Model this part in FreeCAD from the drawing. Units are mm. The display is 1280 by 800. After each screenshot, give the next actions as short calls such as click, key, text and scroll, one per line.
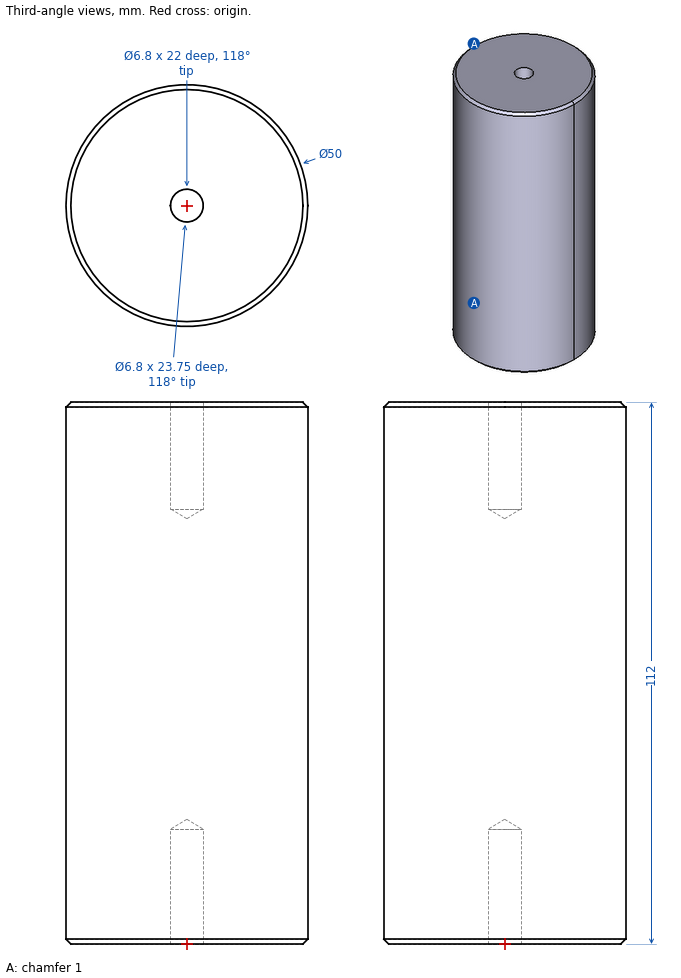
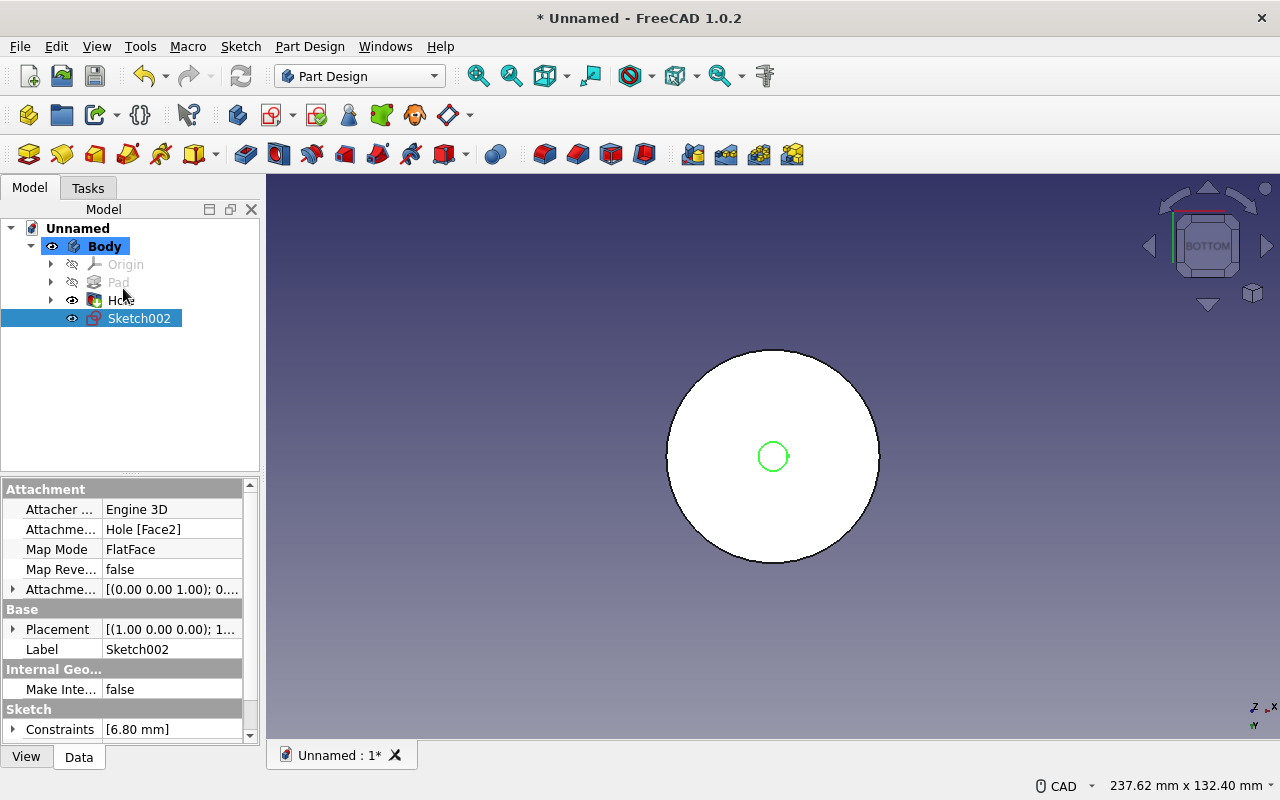
click(279, 154)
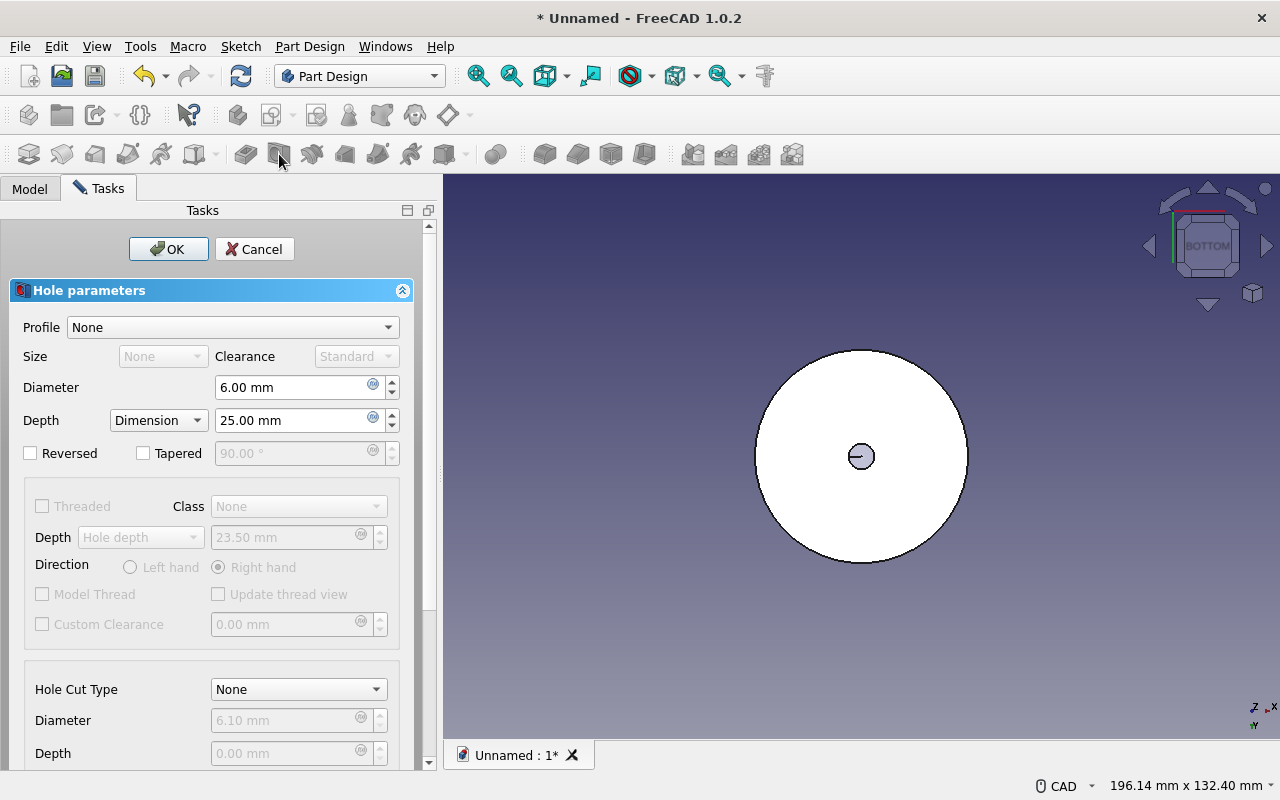
triple_click(300, 388)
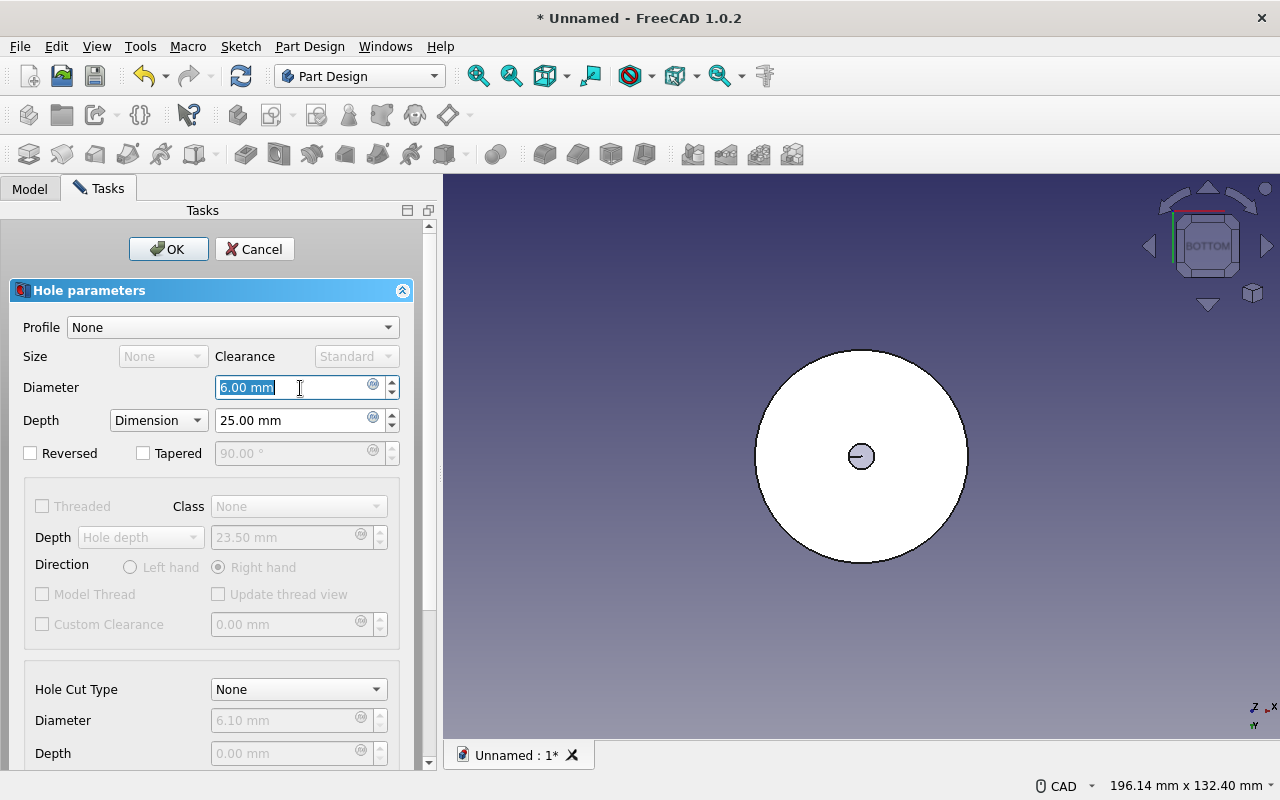
text(6.8)
key(Tab)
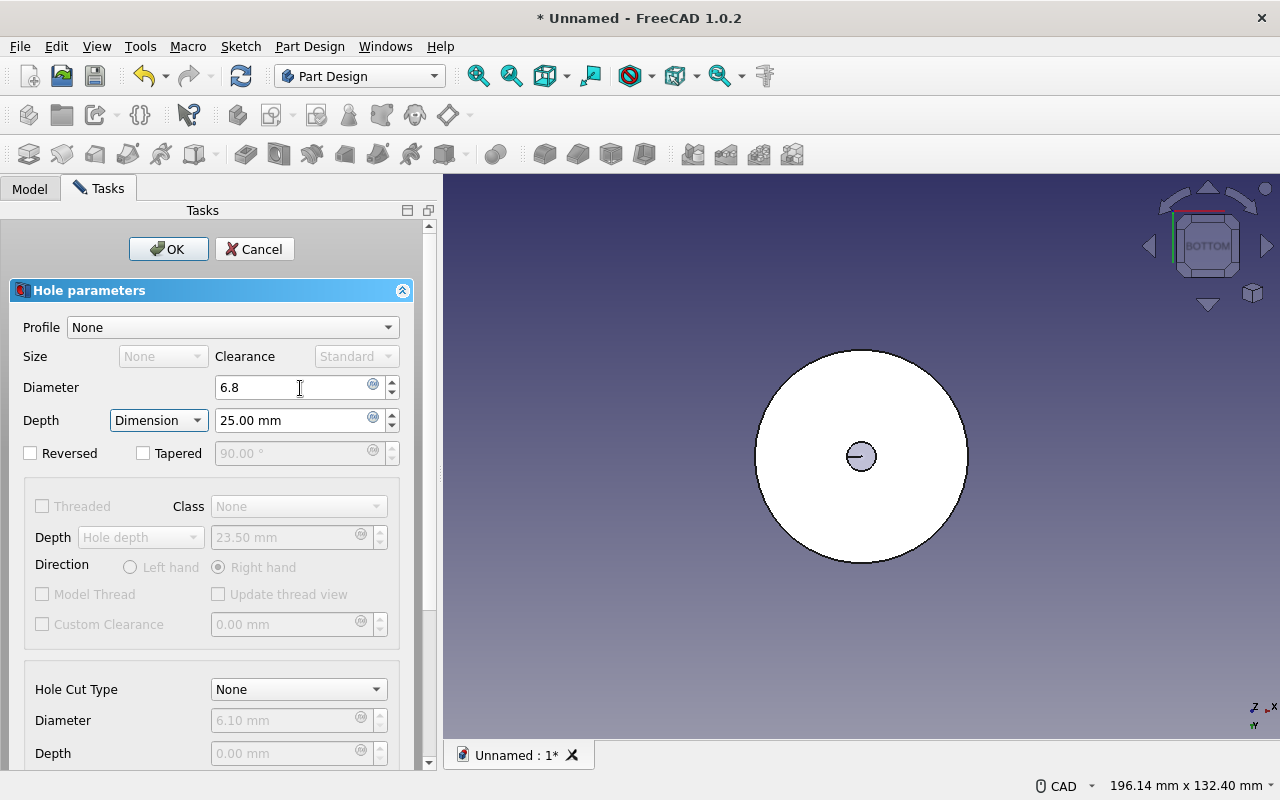
triple_click(300, 420)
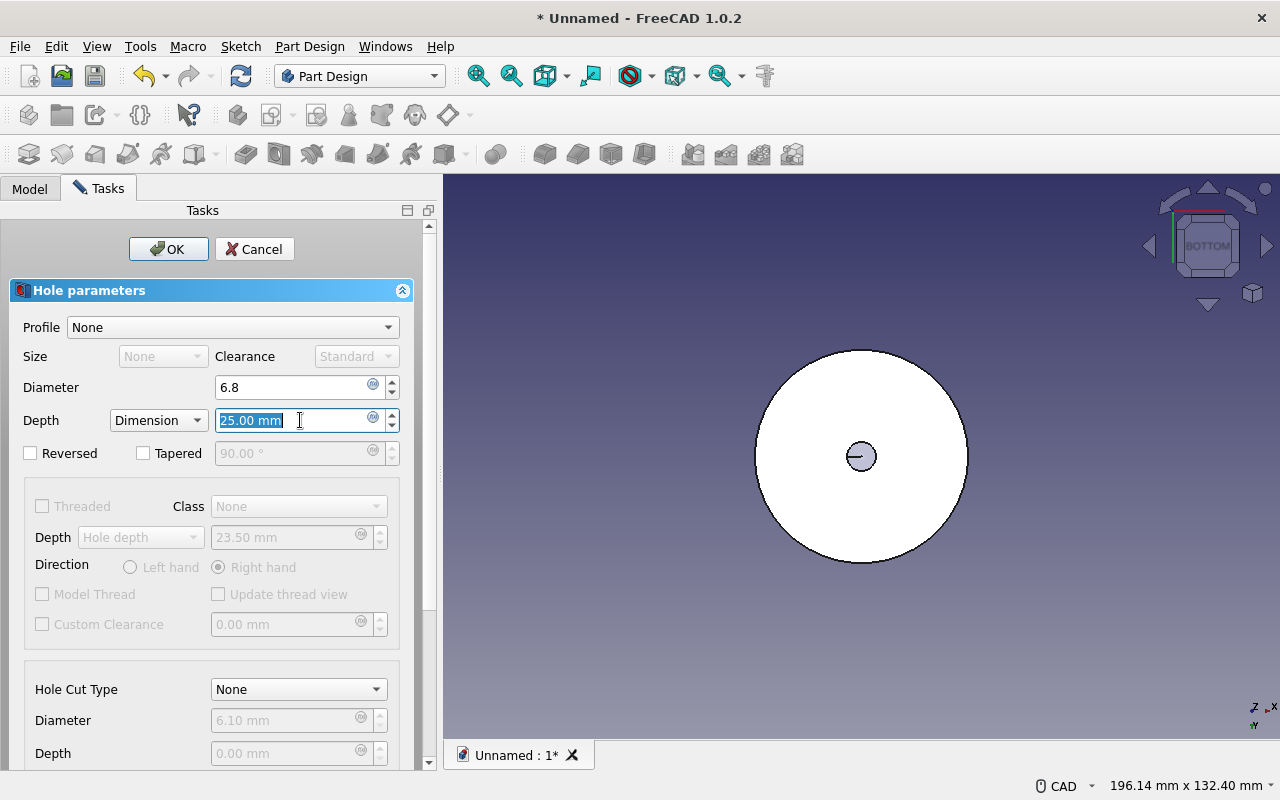
text(23.75)
key(Tab)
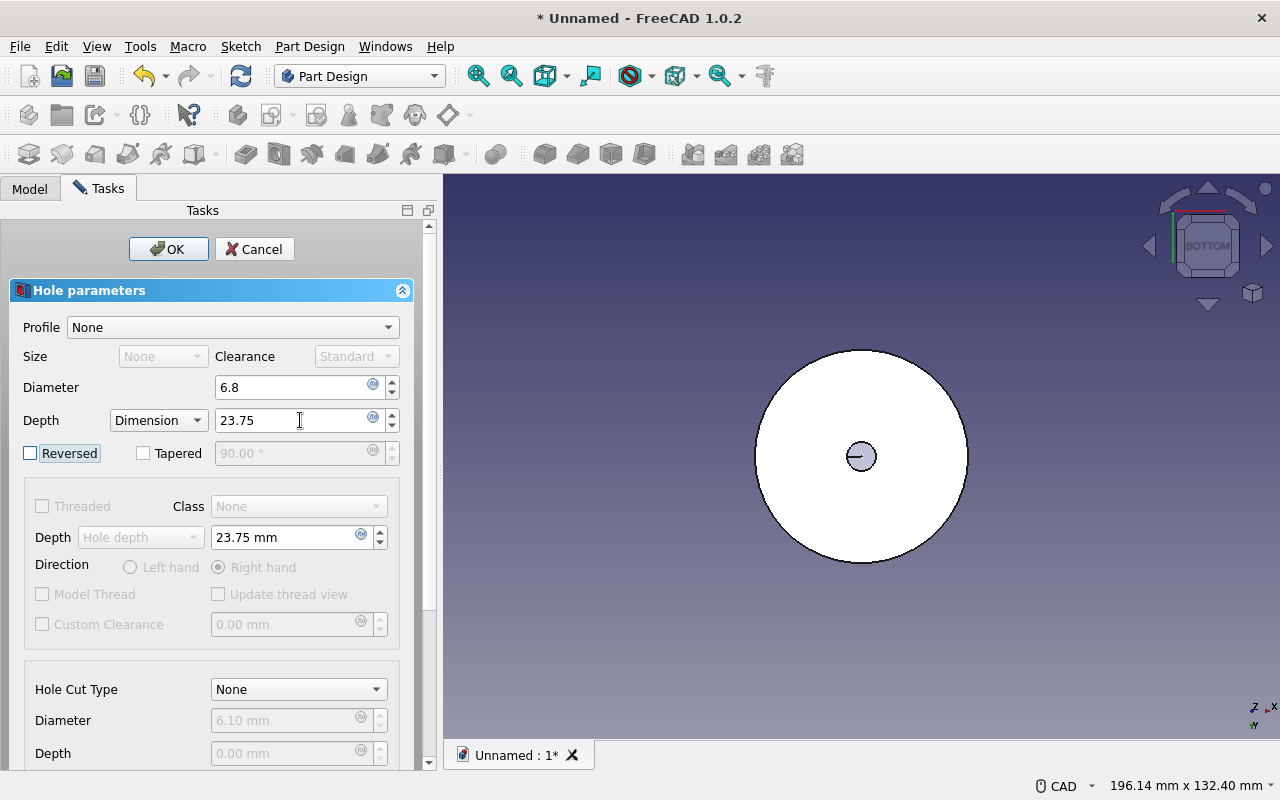
click(169, 249)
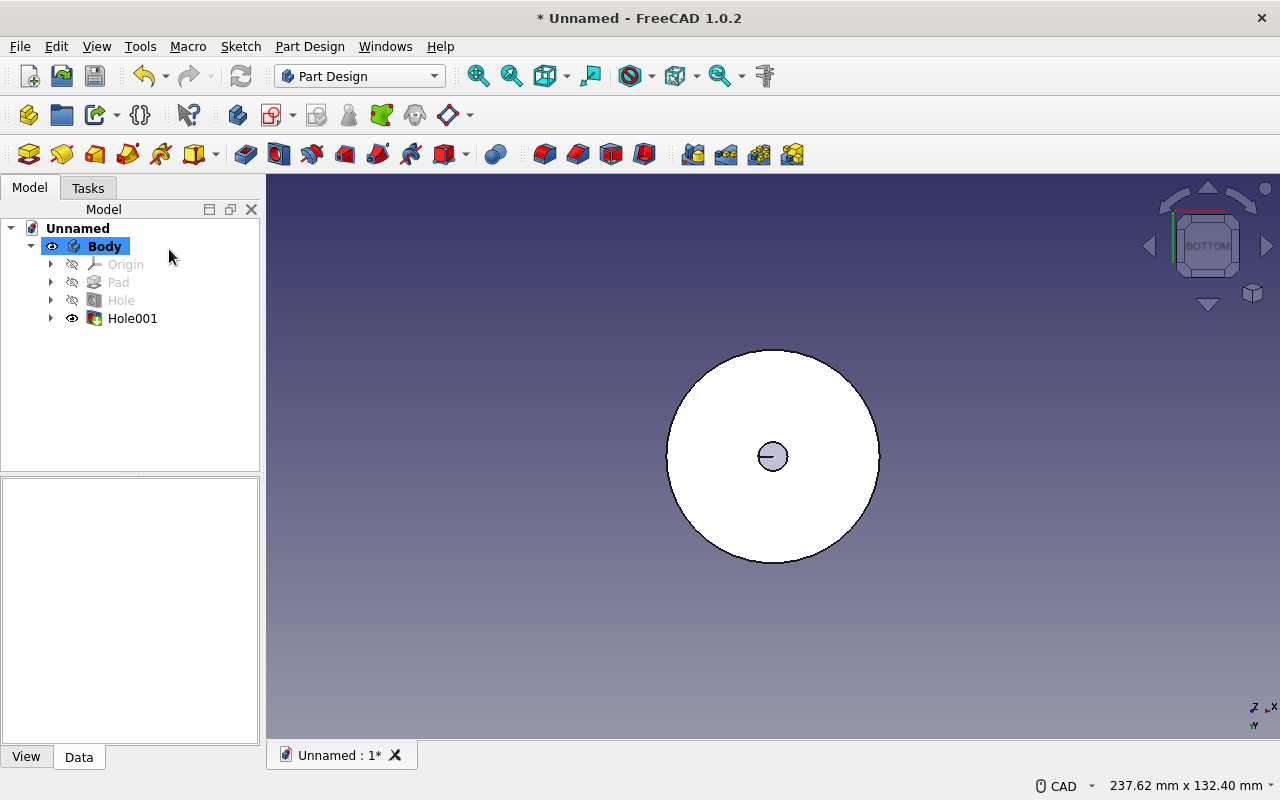
key(v)
key(f)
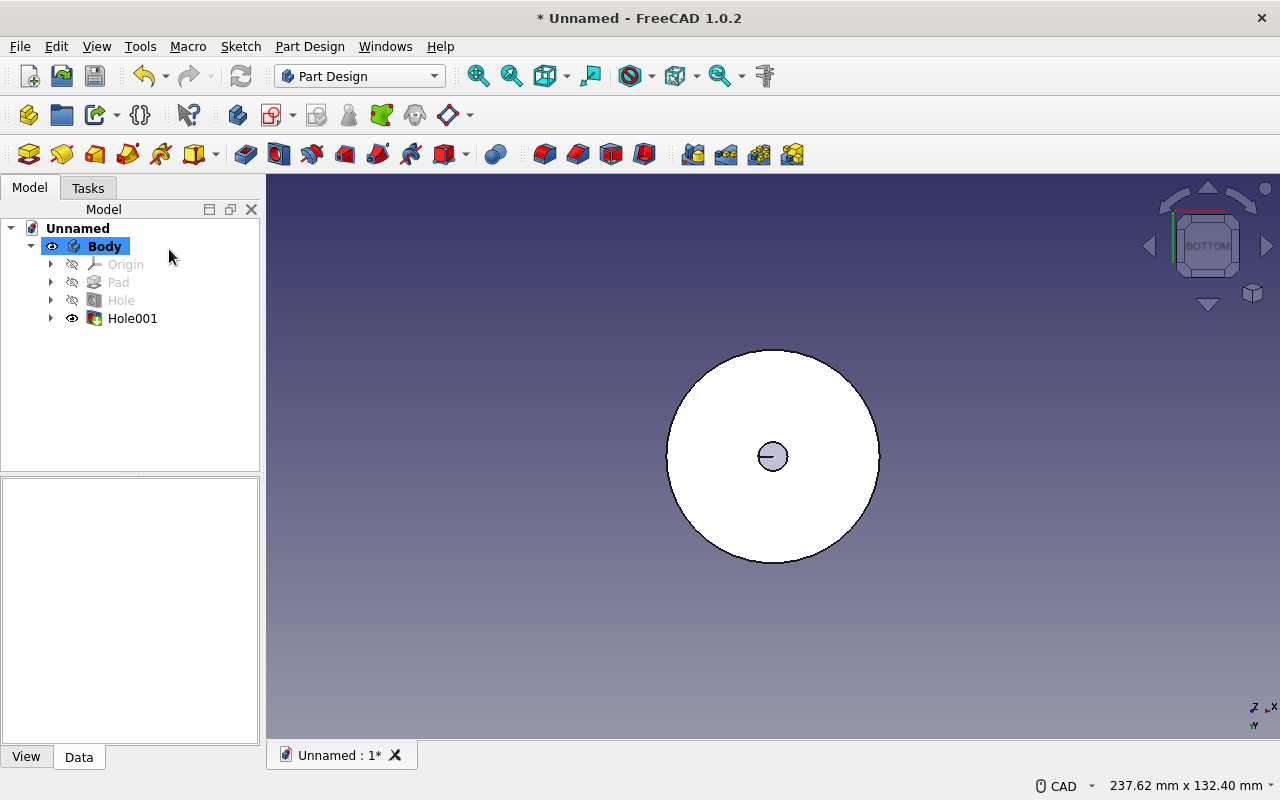
click(666, 455)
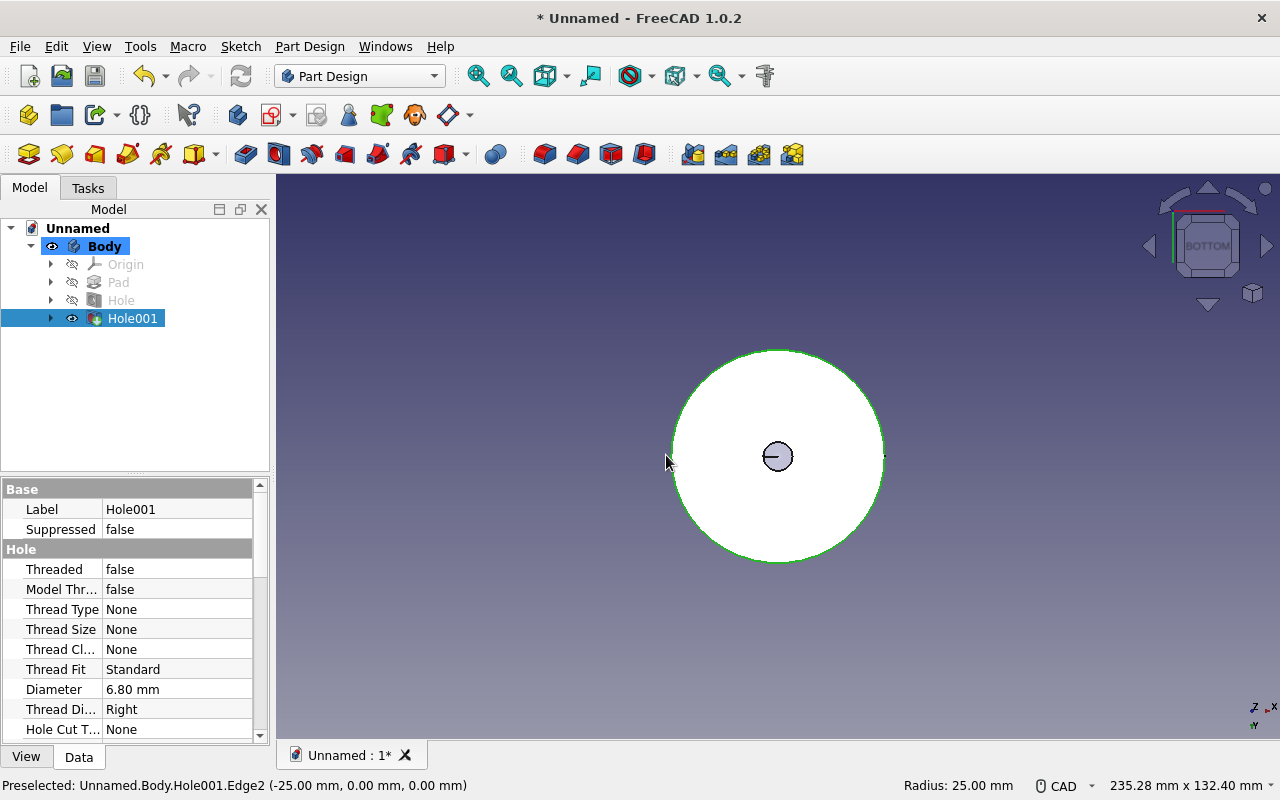
key(0)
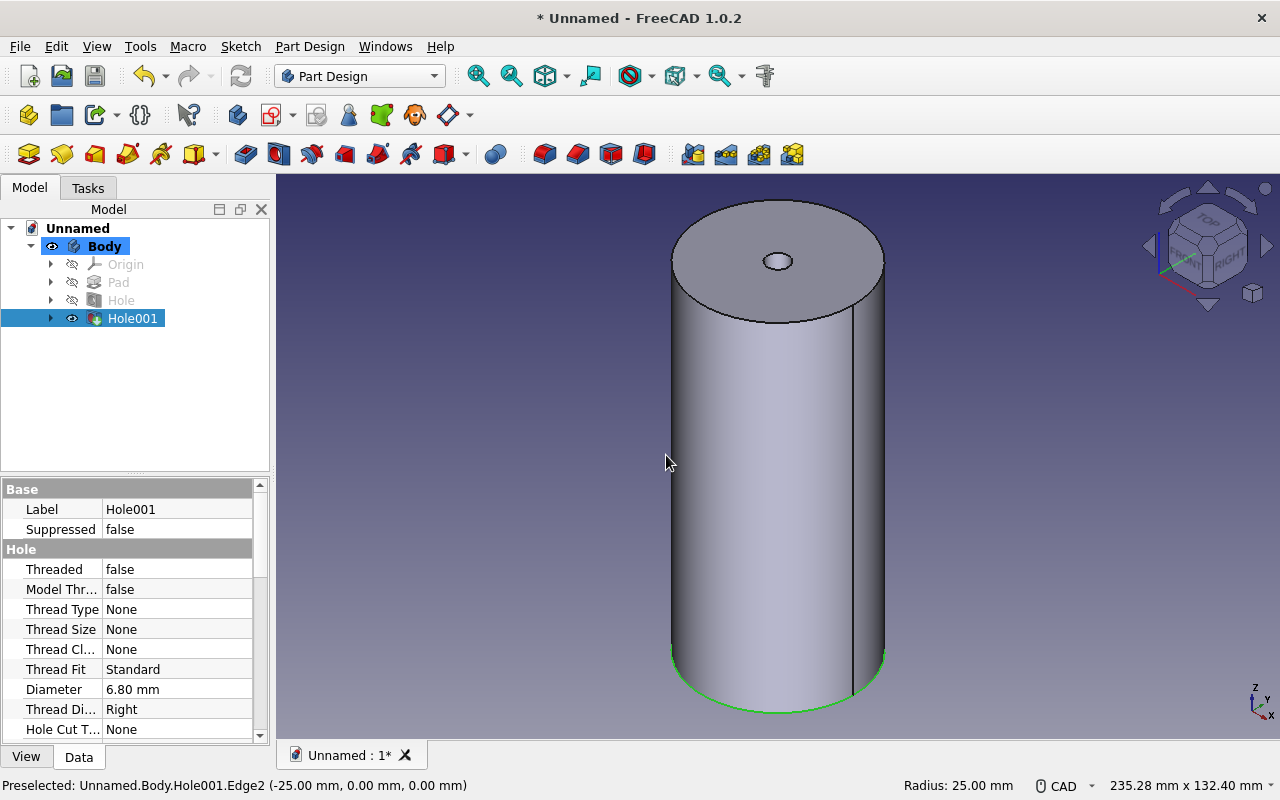
key(v)
key(f)